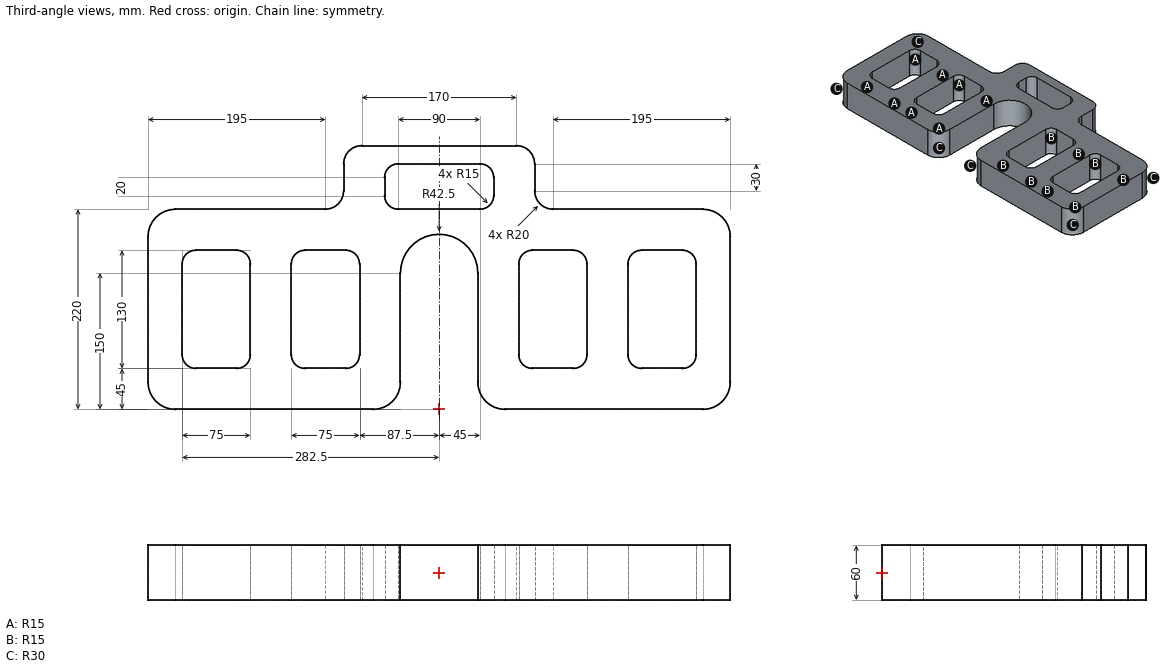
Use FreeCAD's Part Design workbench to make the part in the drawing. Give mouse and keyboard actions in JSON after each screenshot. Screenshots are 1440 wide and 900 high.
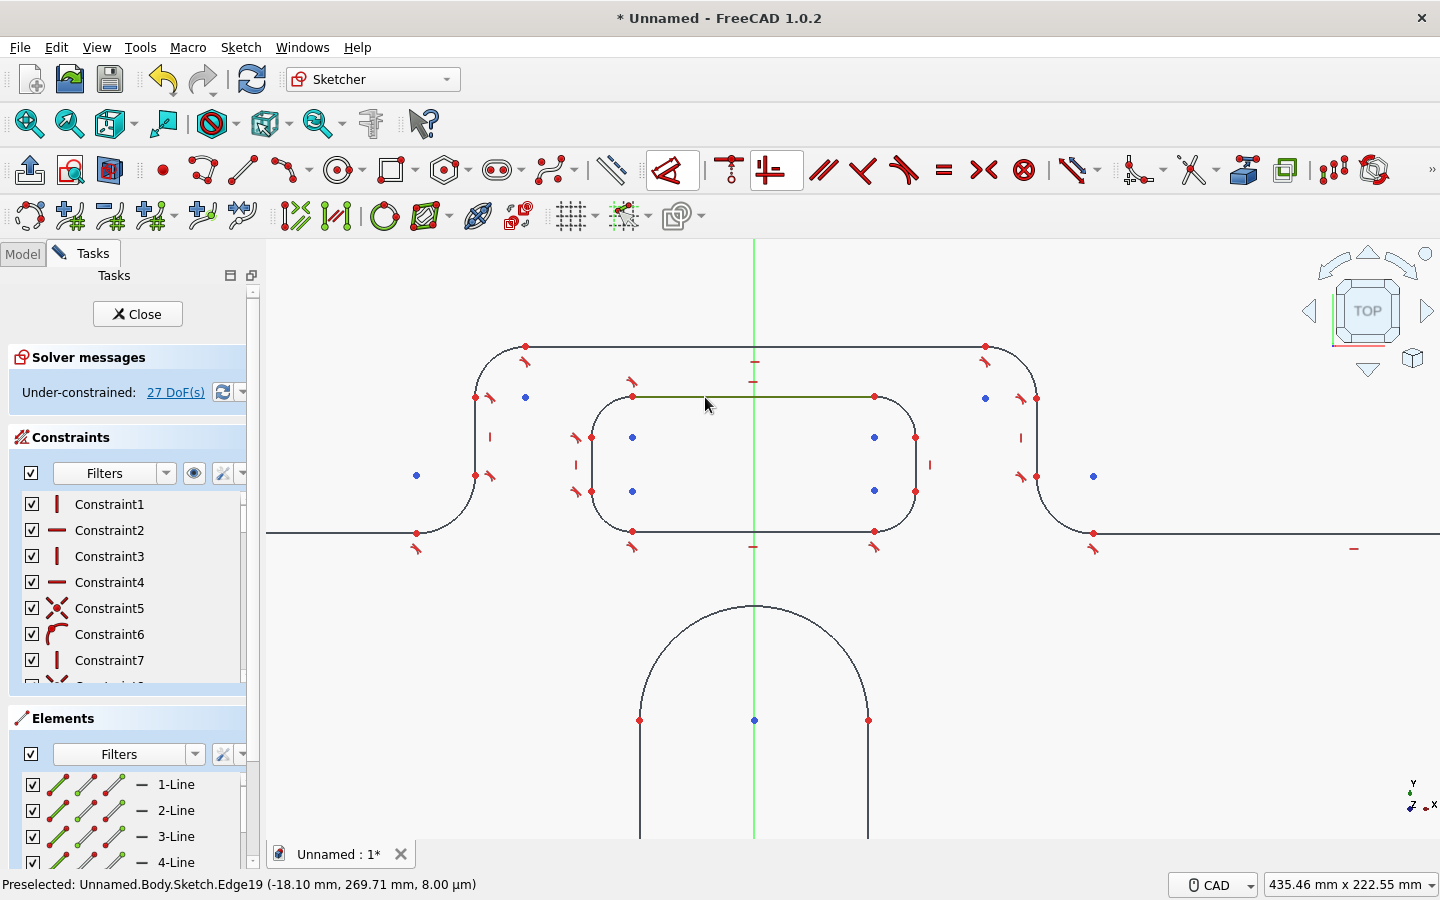
{"action": "left_click", "coordinate": [911, 419]}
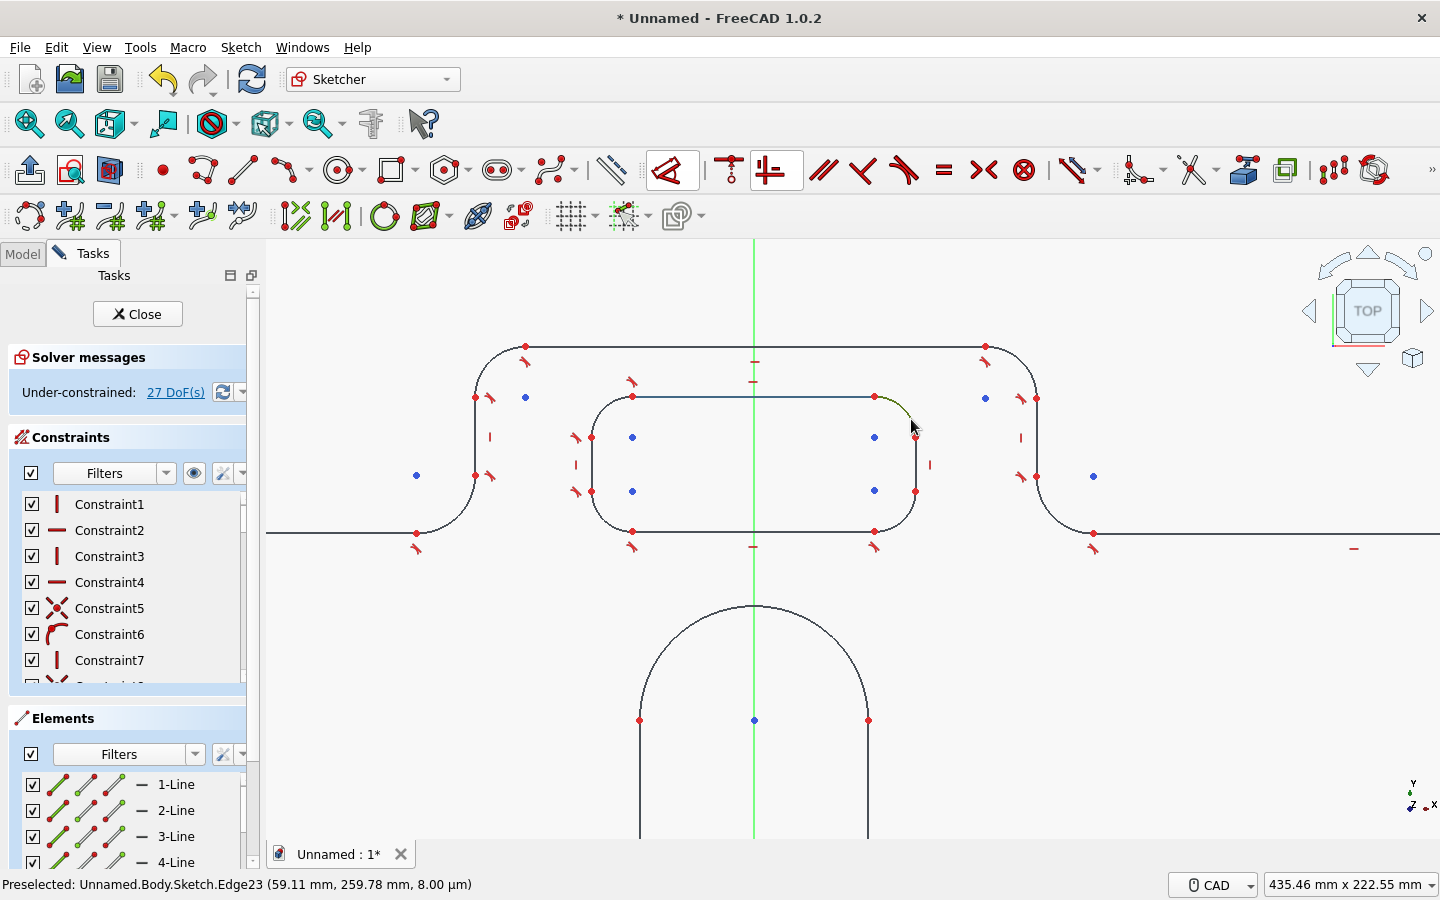
{"action": "left_click", "coordinate": [904, 170]}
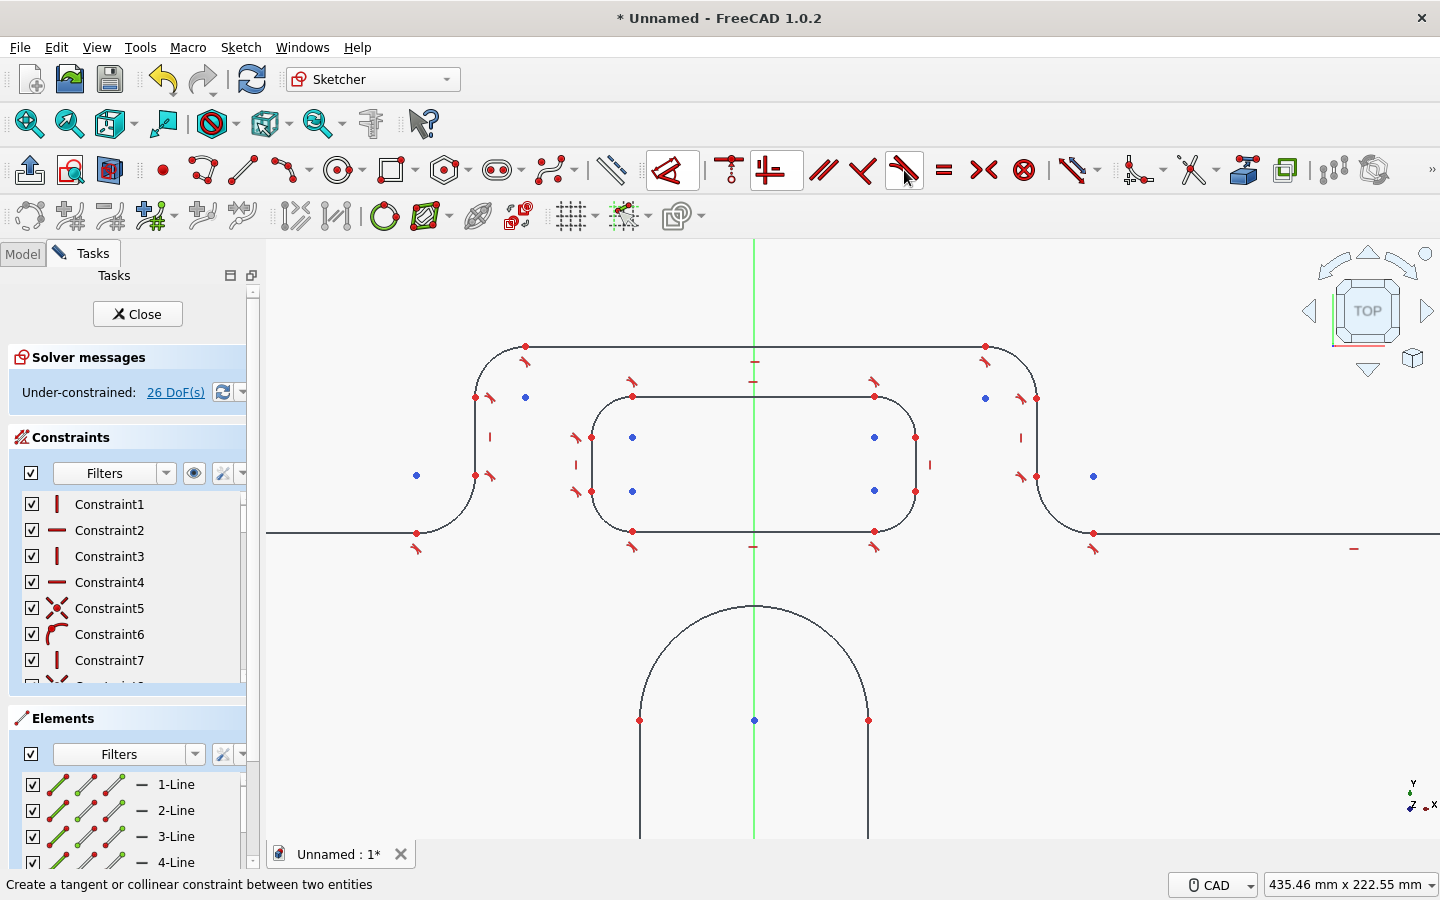
{"action": "left_click", "coordinate": [916, 453]}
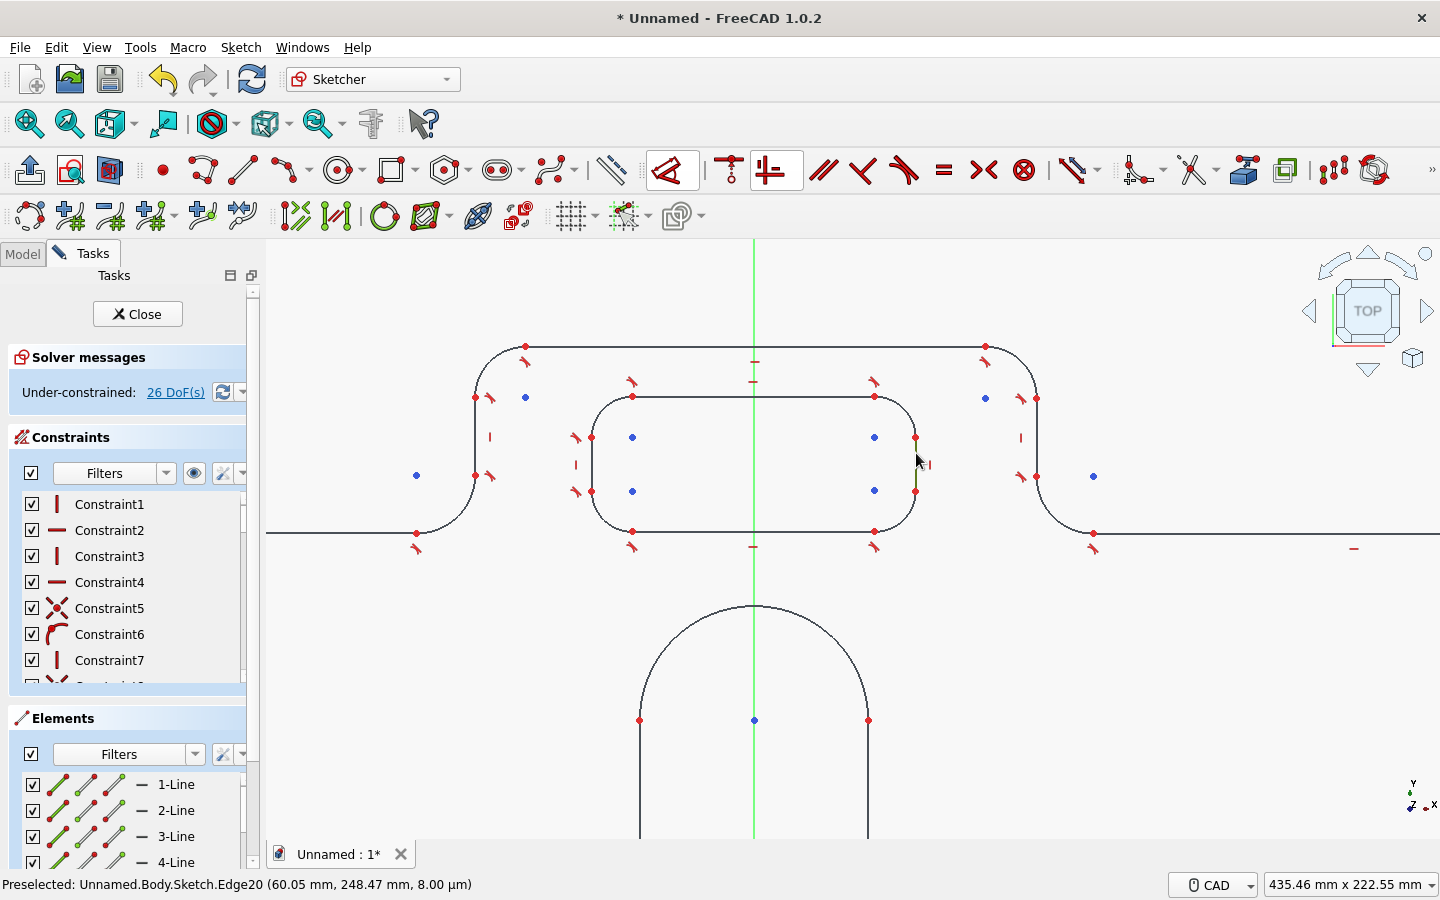
{"action": "left_click", "coordinate": [911, 419]}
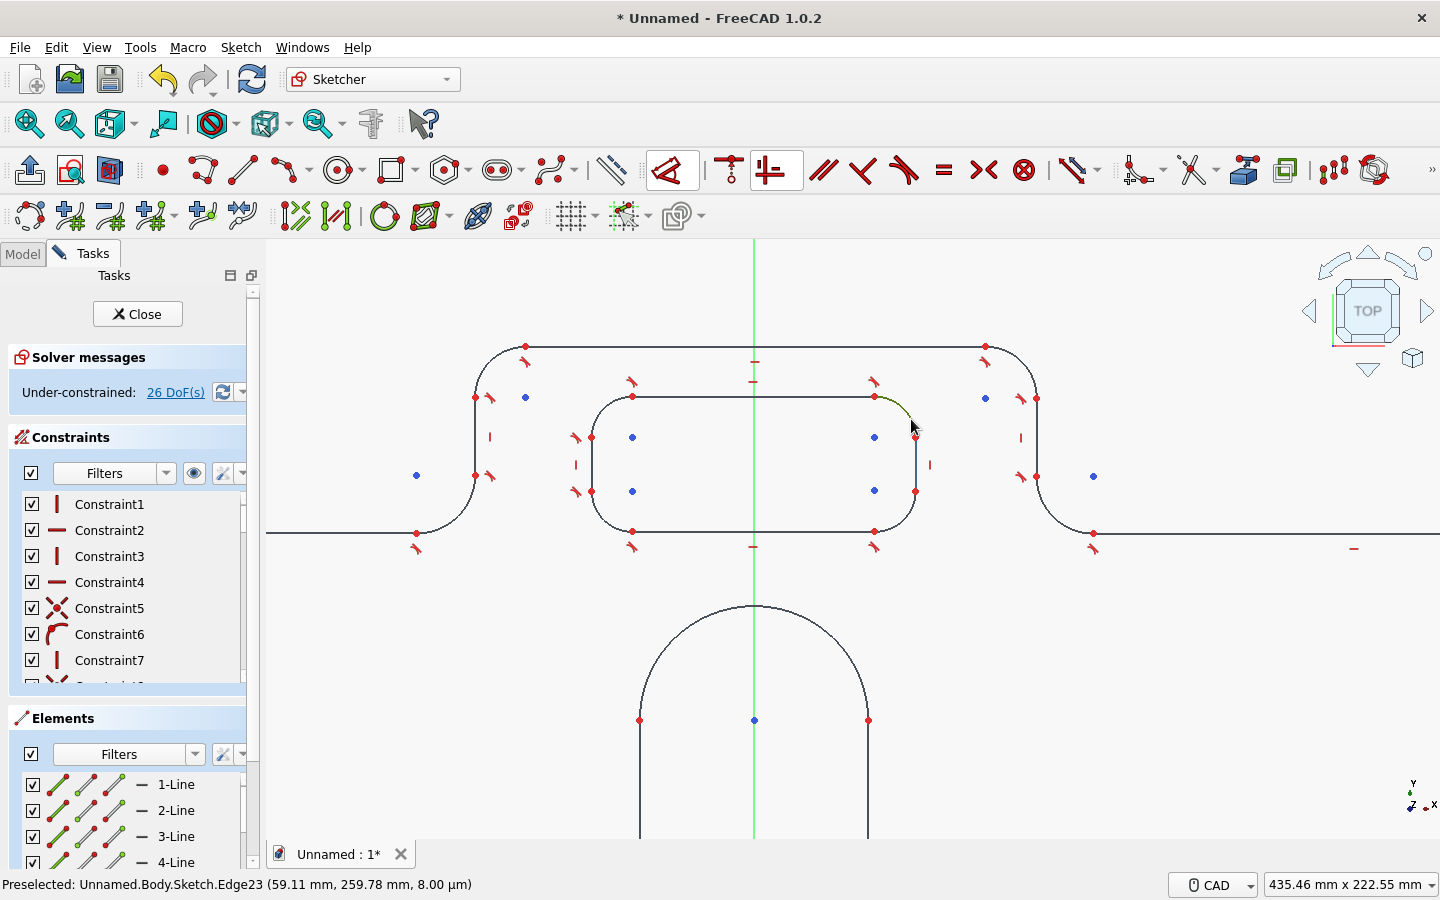
{"action": "left_click", "coordinate": [904, 170]}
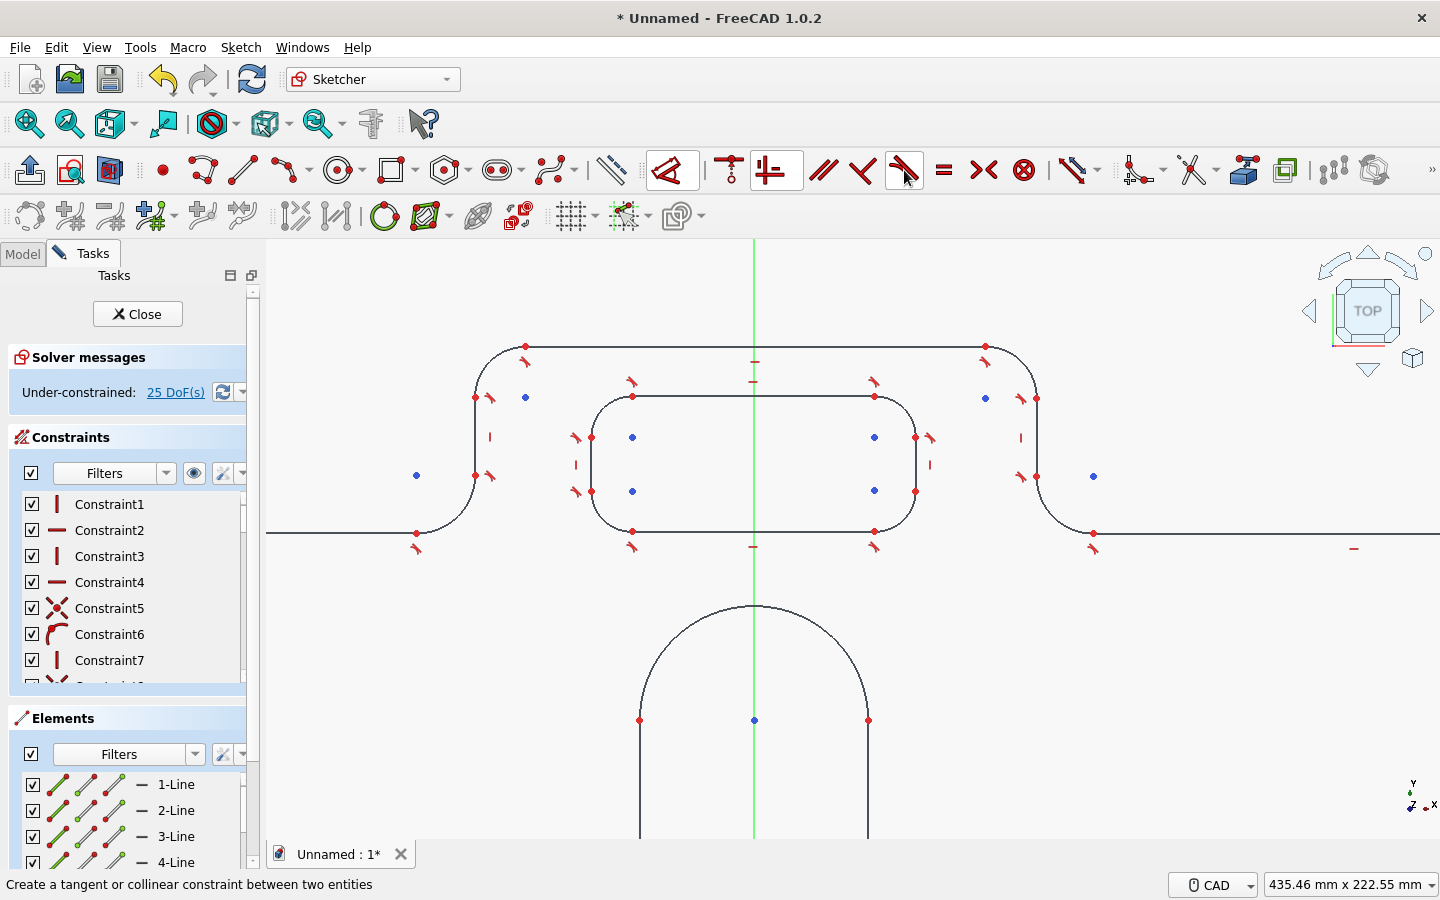
{"action": "left_click", "coordinate": [916, 453]}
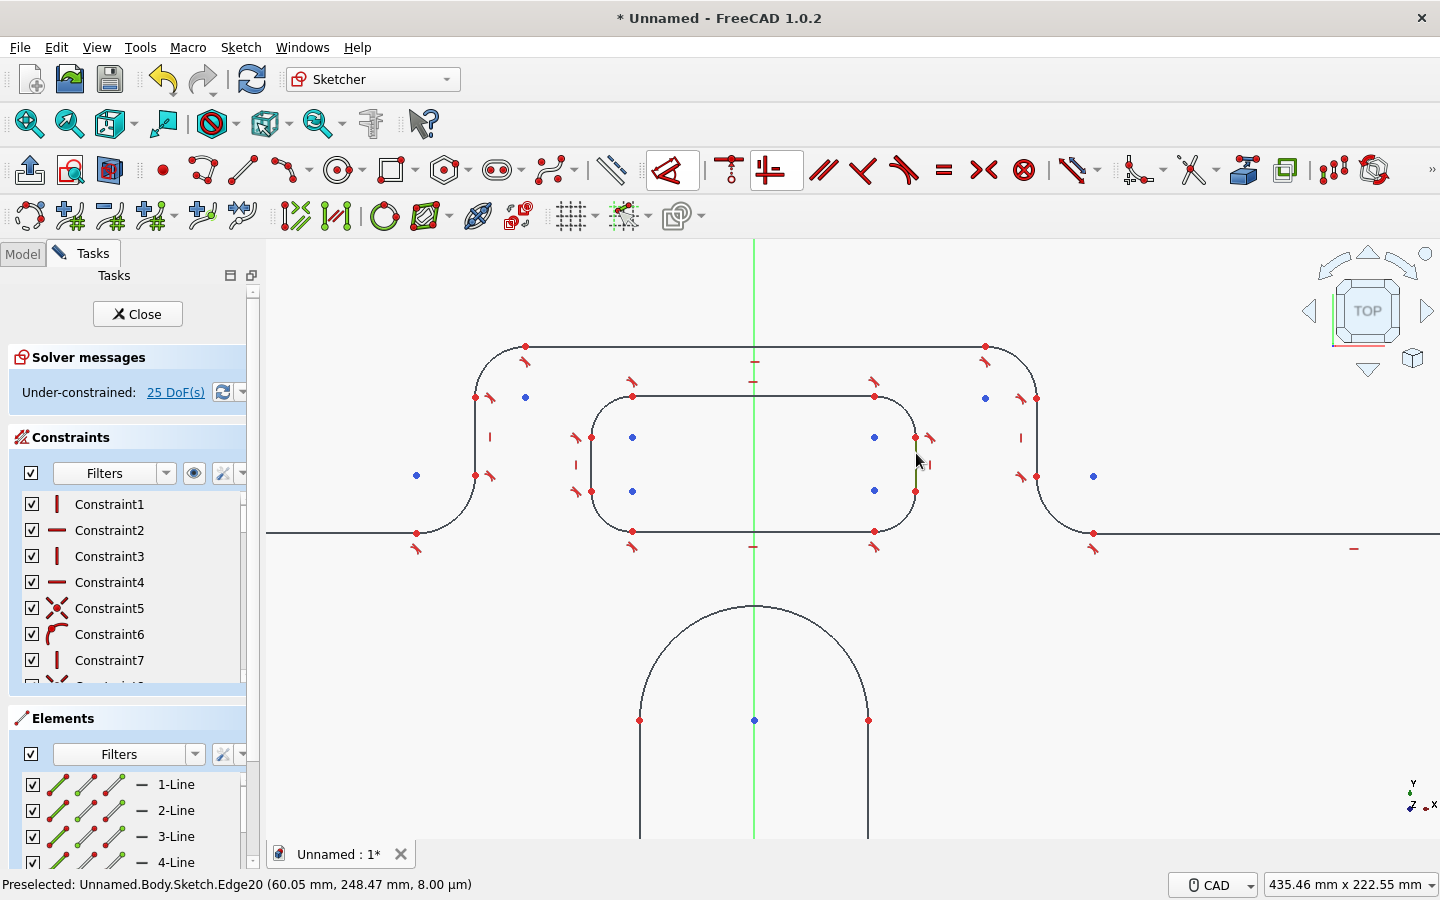
{"action": "left_click", "coordinate": [893, 527]}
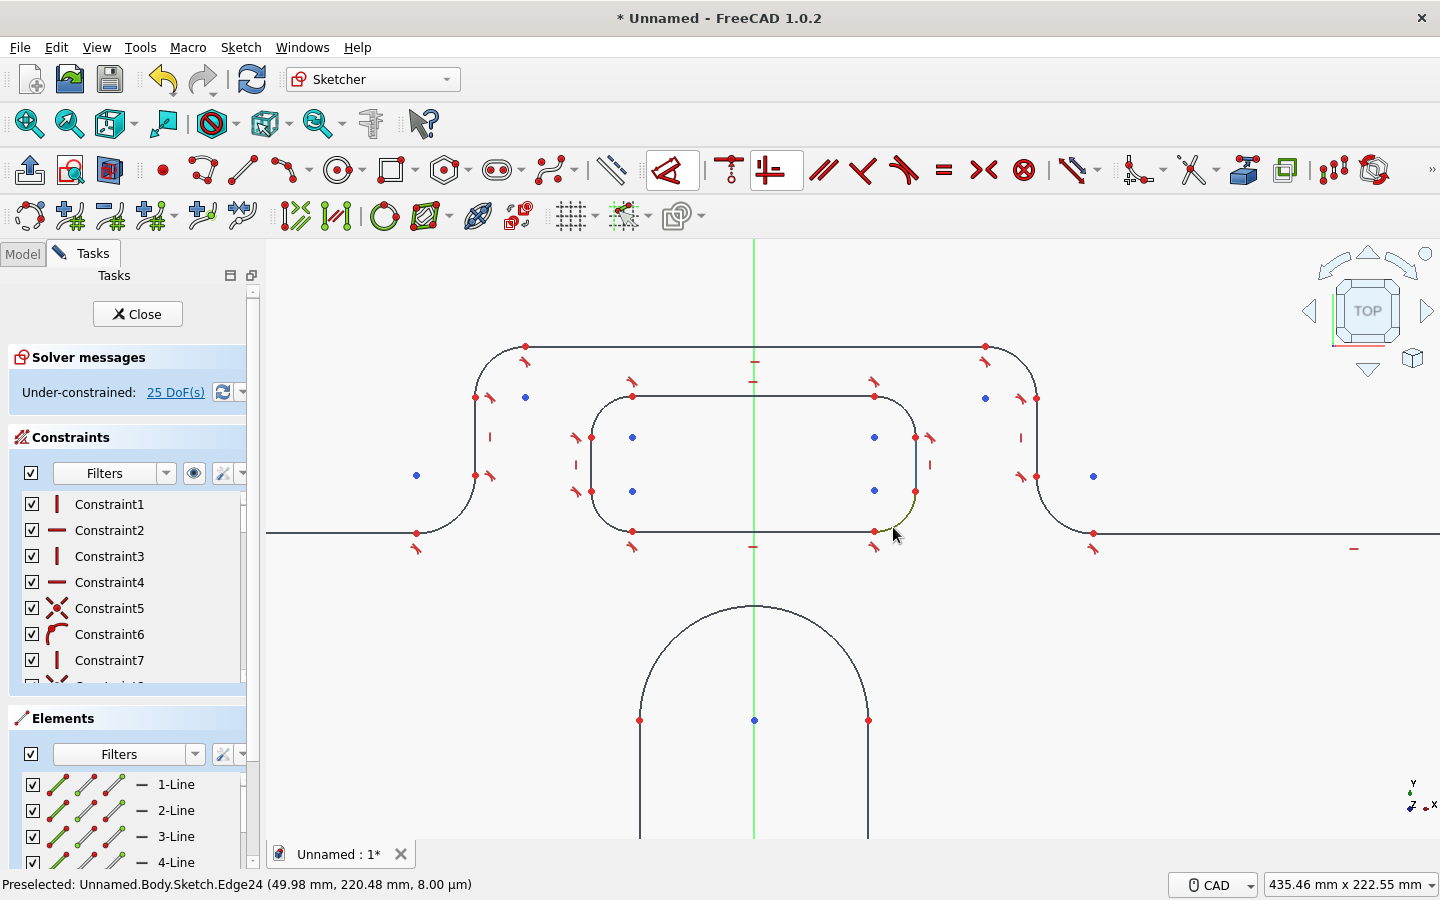
{"action": "left_click", "coordinate": [904, 170]}